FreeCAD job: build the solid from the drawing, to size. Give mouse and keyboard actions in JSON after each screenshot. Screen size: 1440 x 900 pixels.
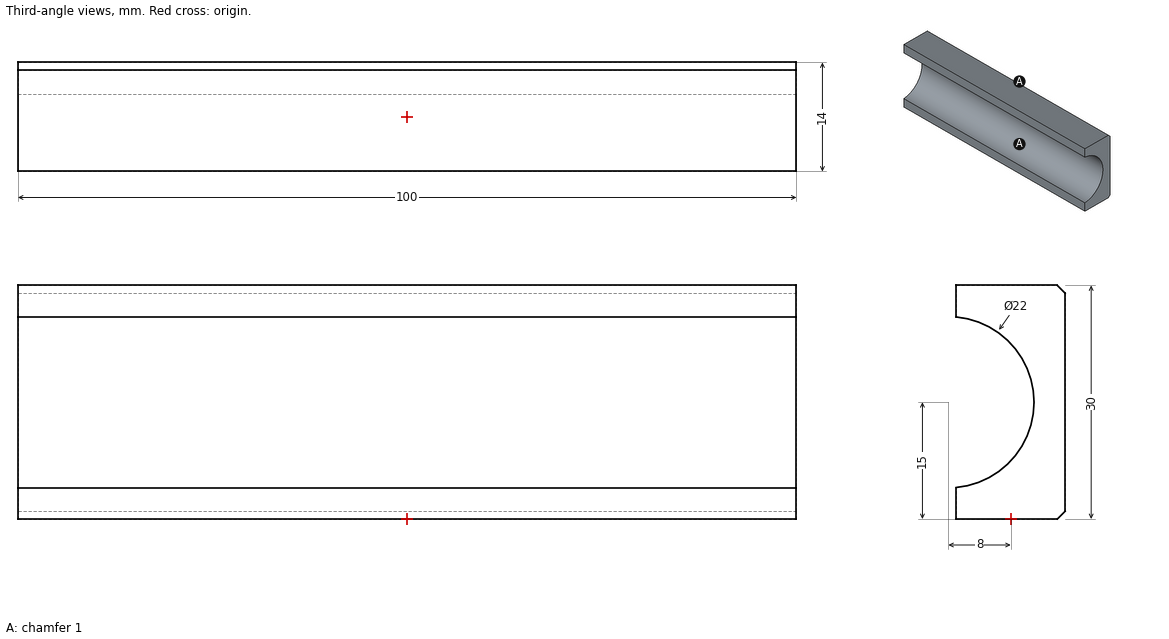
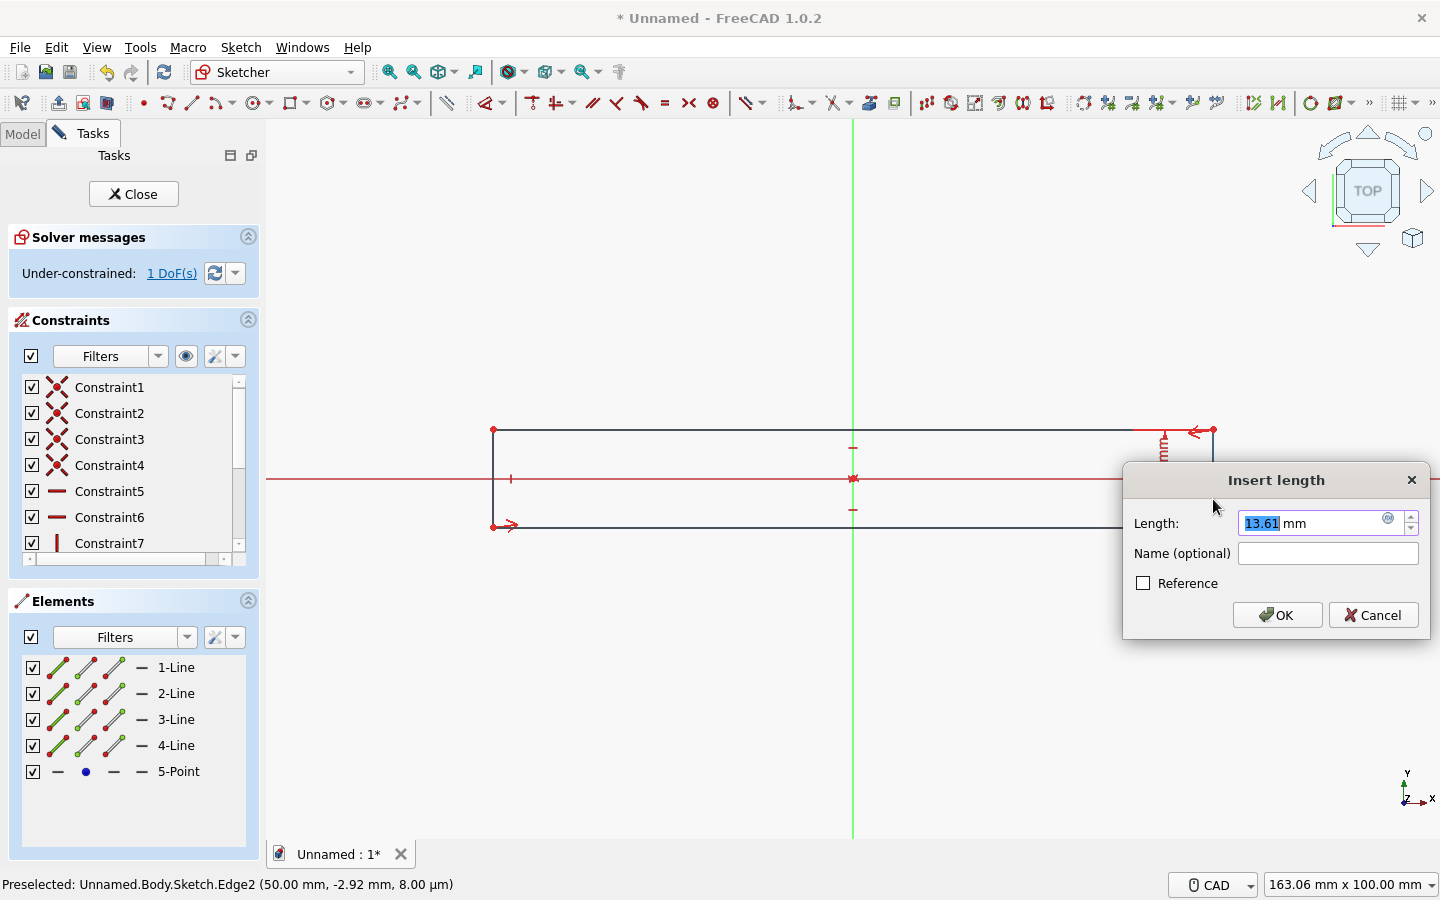
{"action": "type", "text": "14"}
{"action": "key", "text": "Return"}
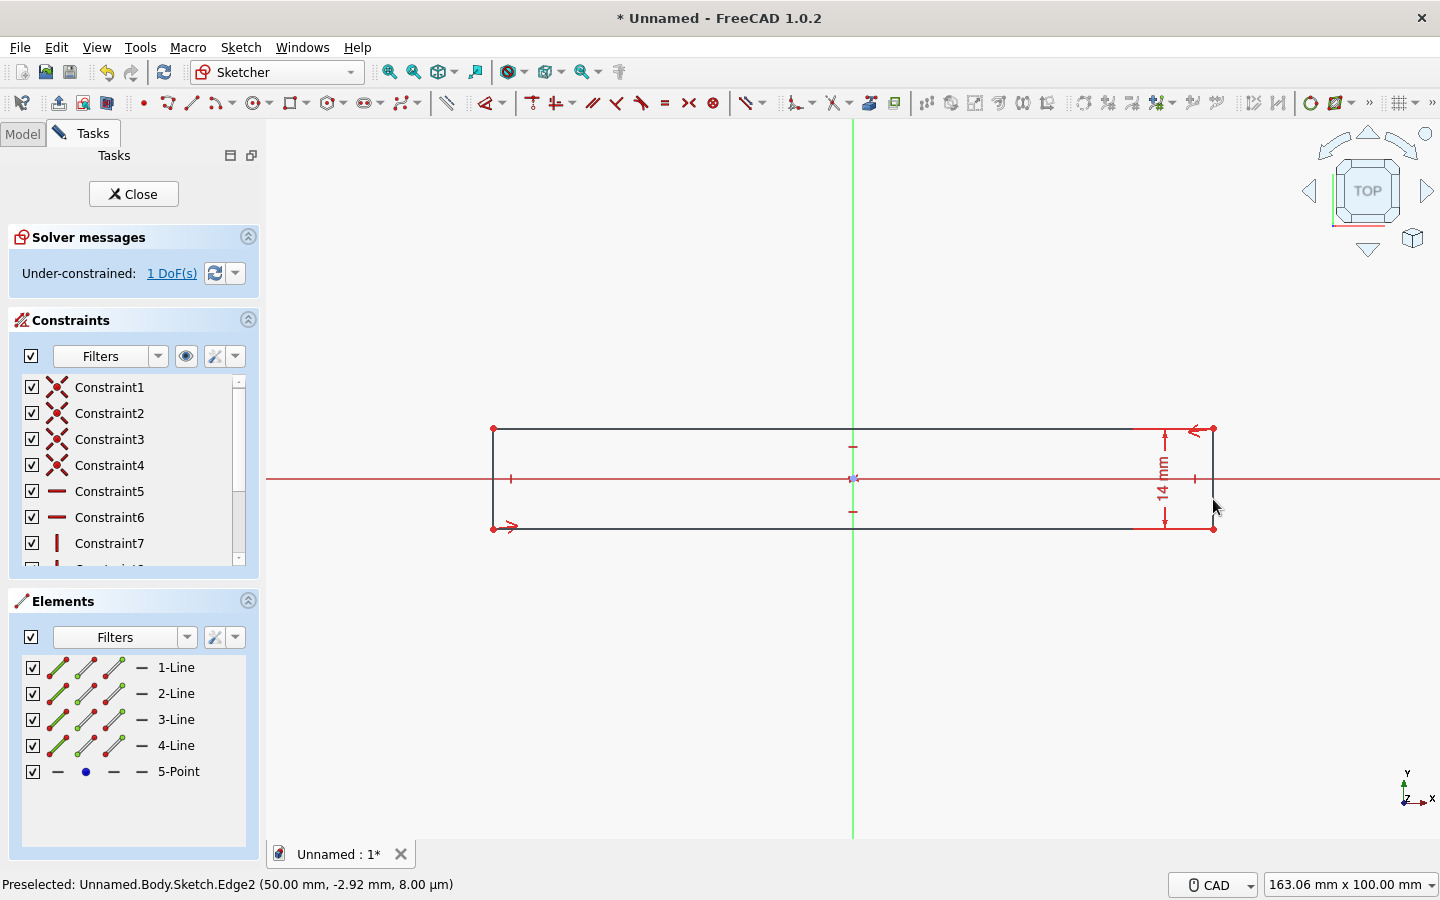
{"action": "left_click", "coordinate": [709, 529]}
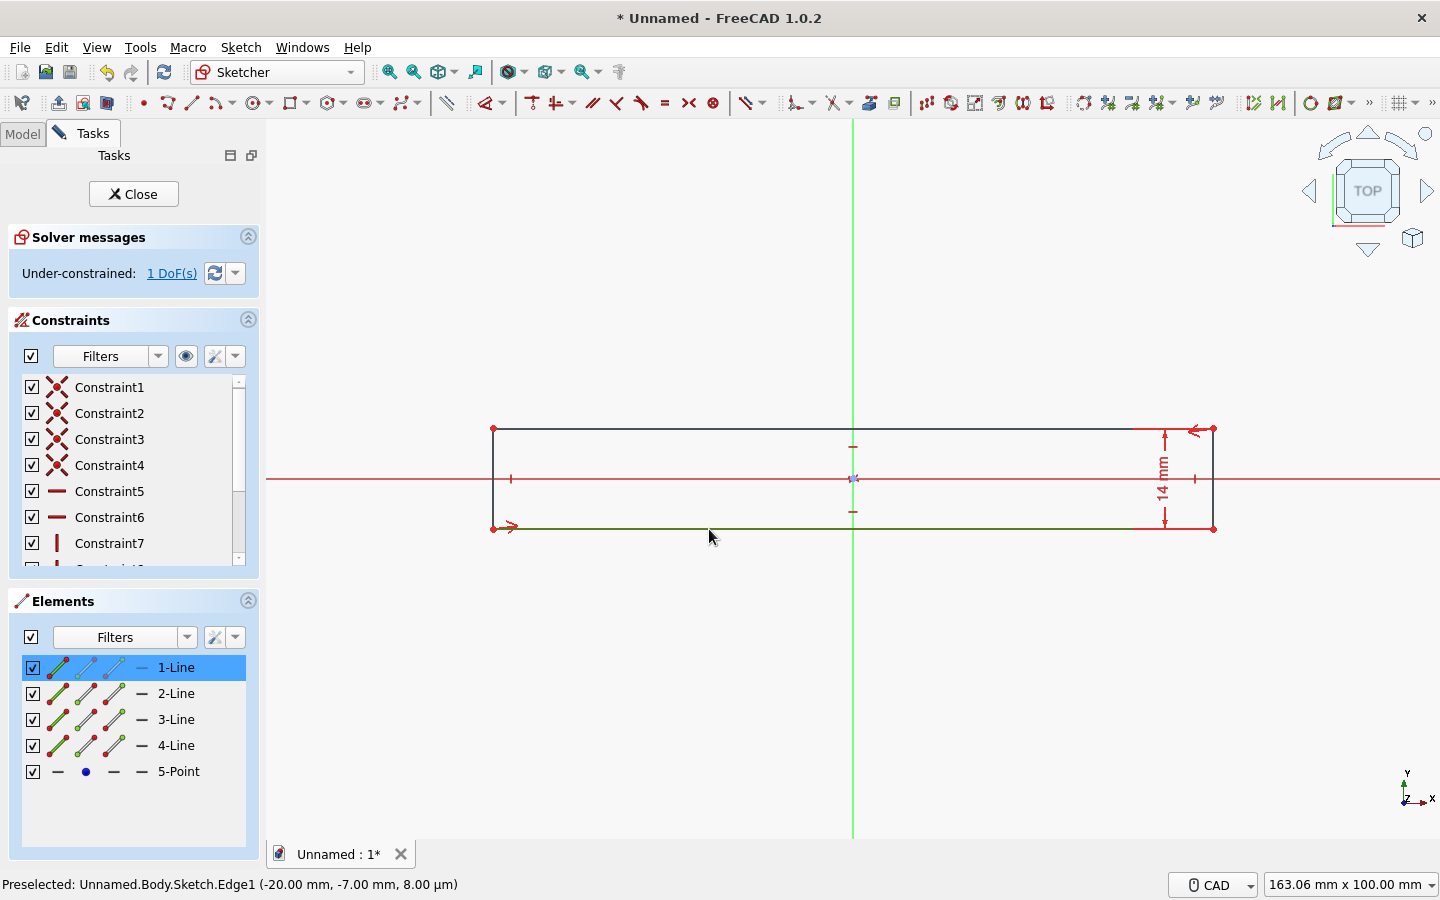
{"action": "left_click", "coordinate": [504, 104]}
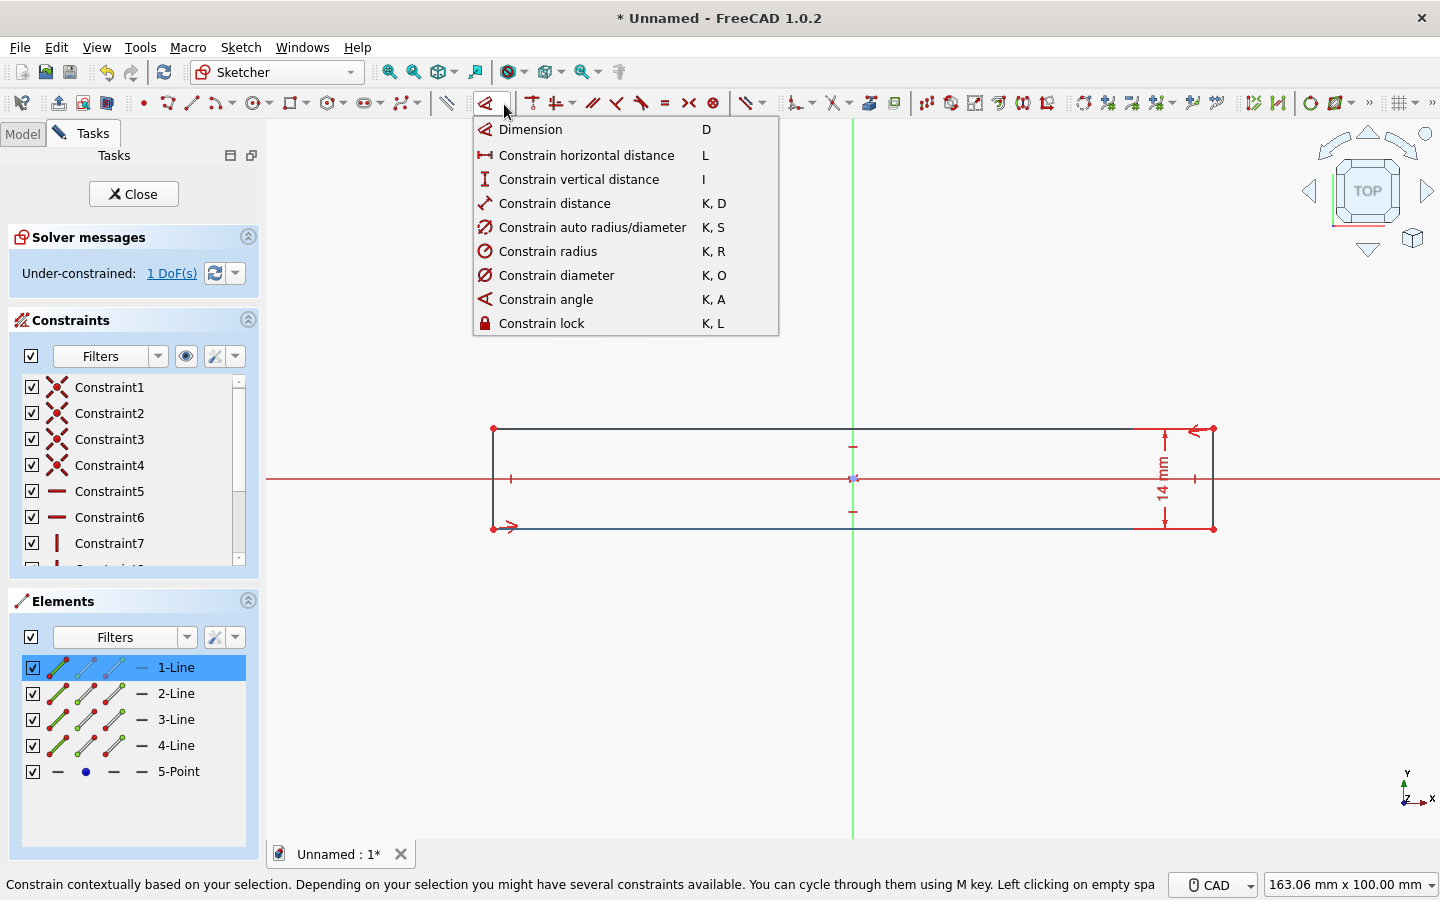
{"action": "left_click", "coordinate": [626, 155]}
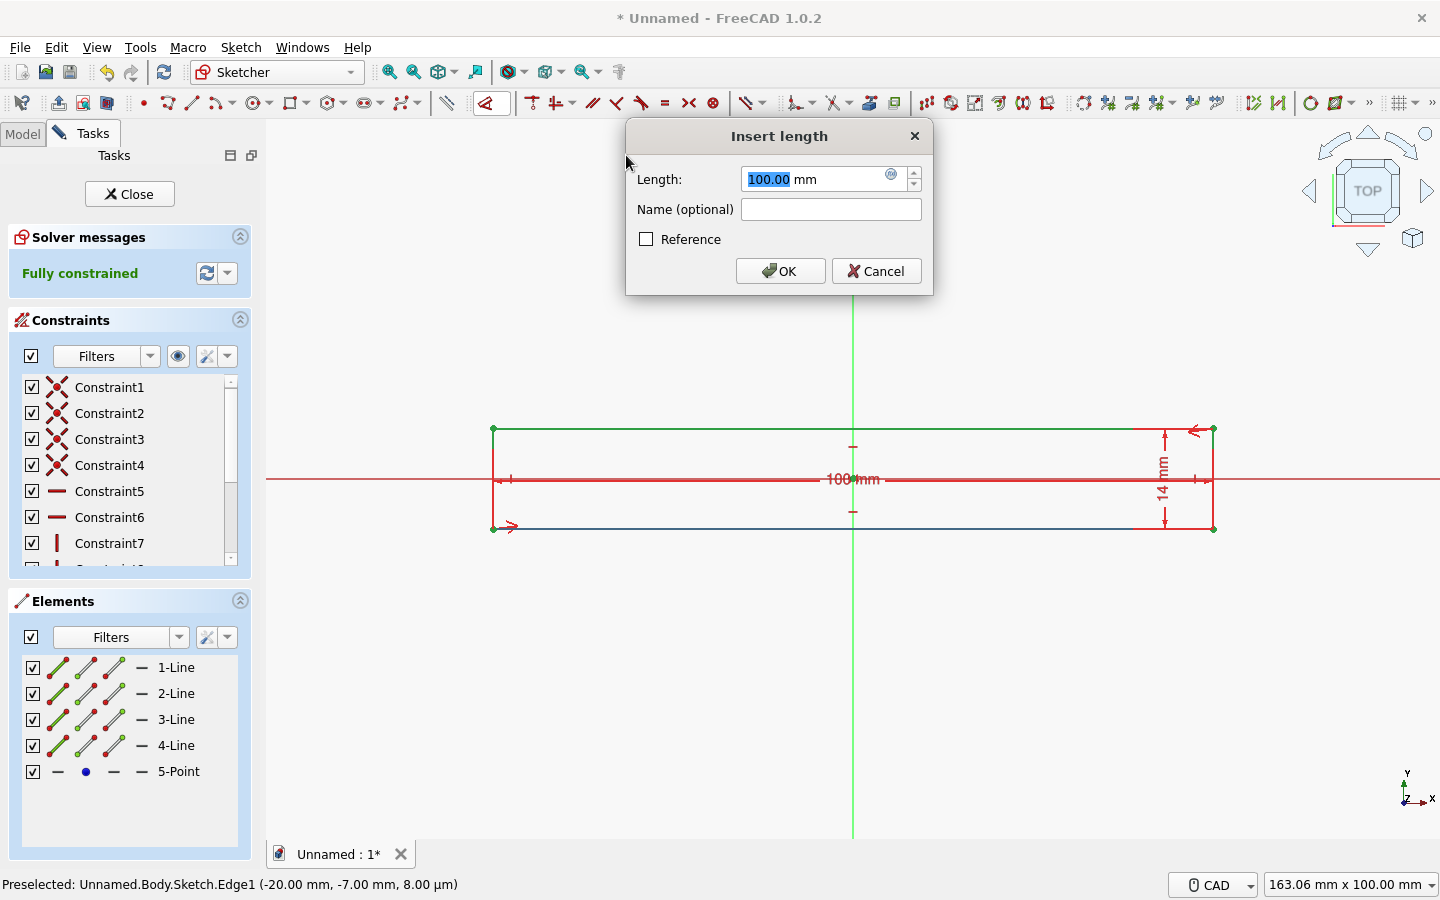
{"action": "type", "text": "100"}
{"action": "key", "text": "Return"}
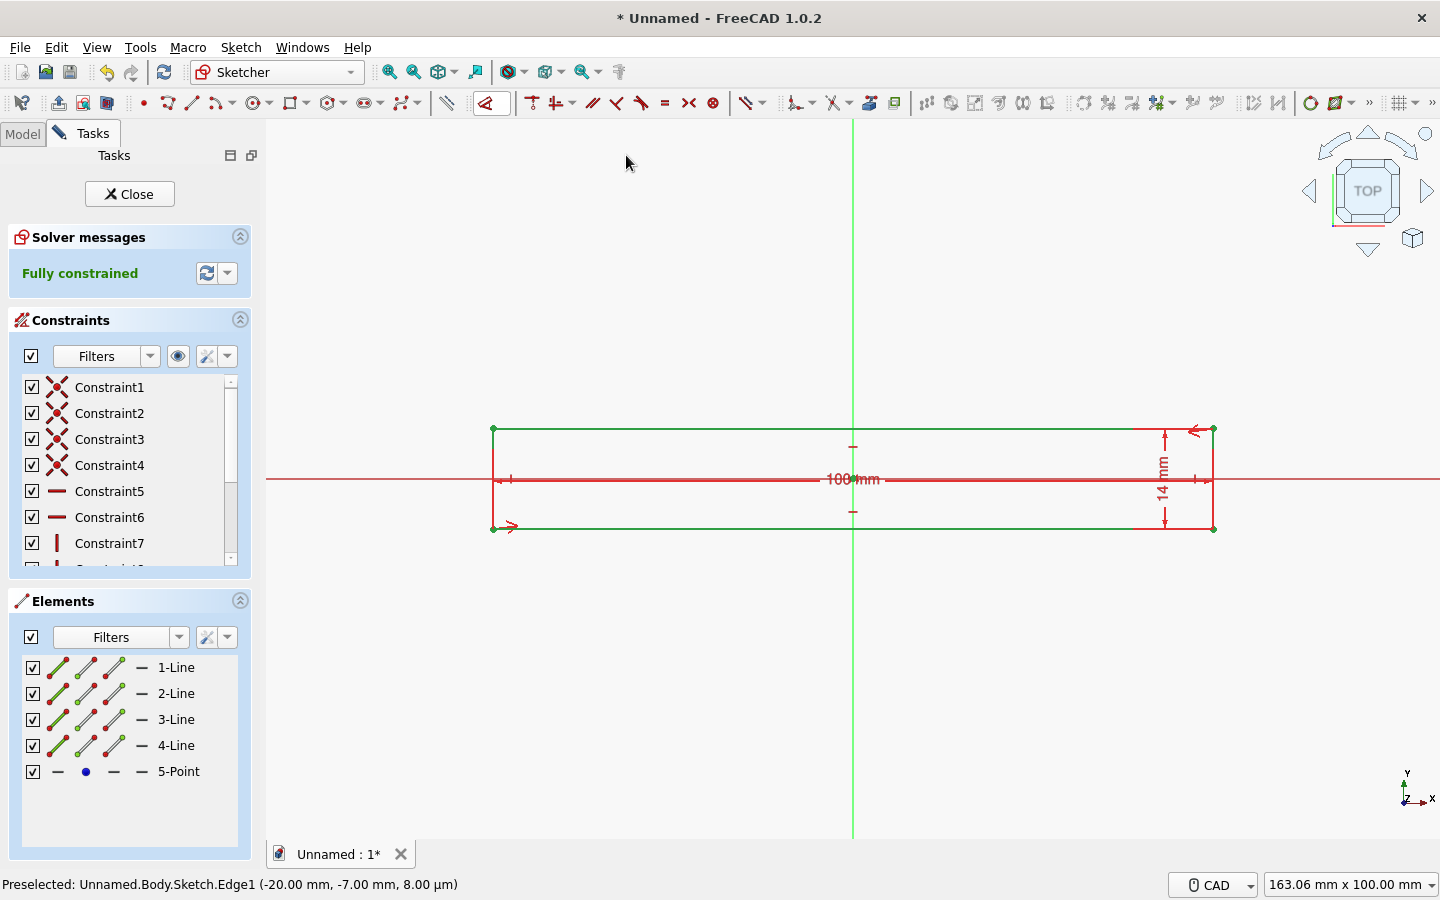
{"action": "left_click", "coordinate": [130, 194]}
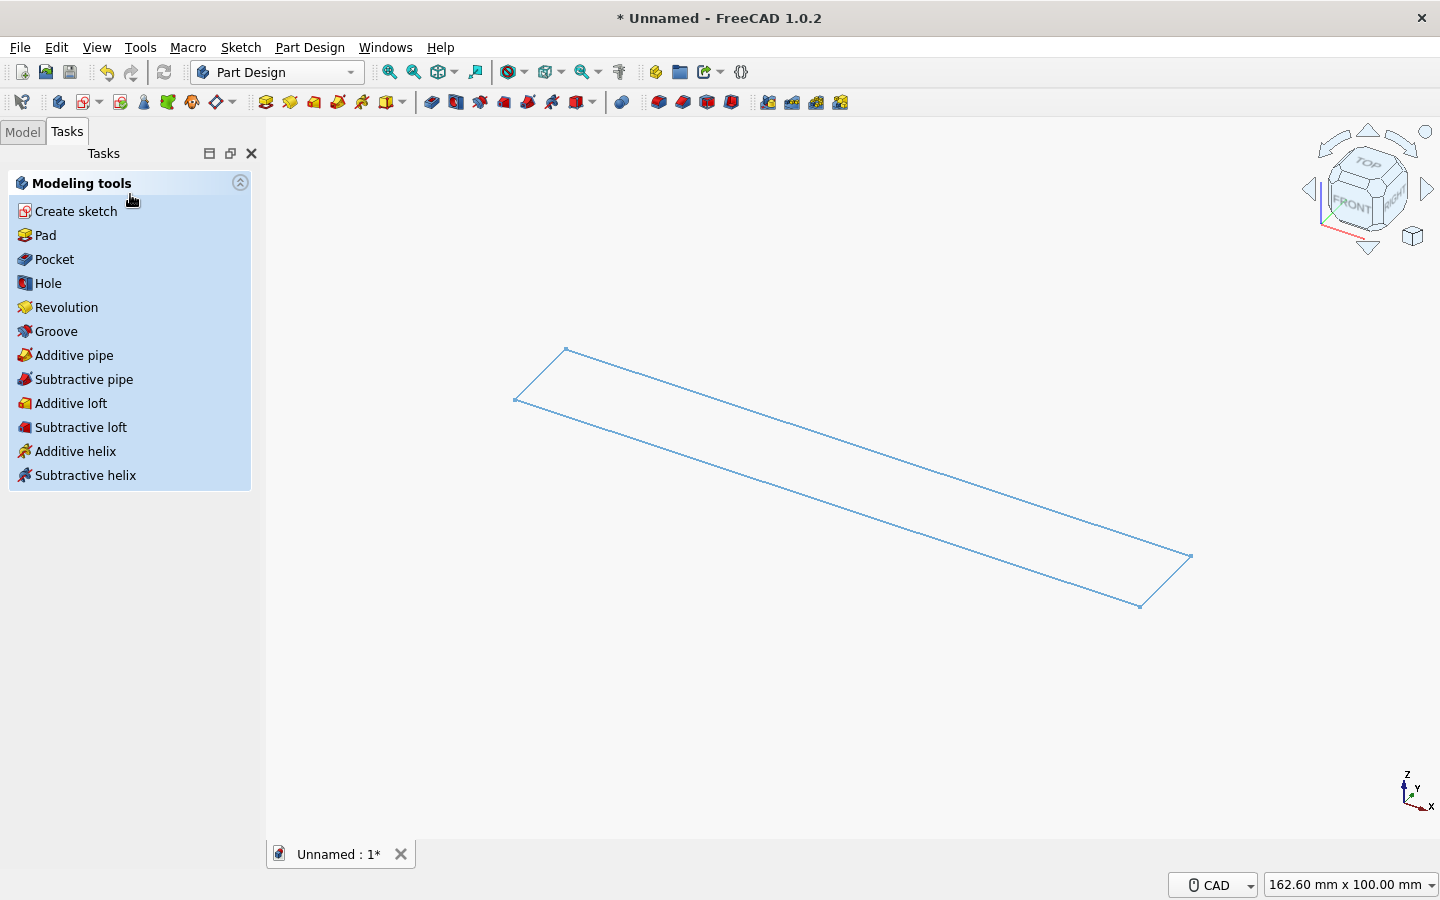
{"action": "left_click", "coordinate": [266, 102]}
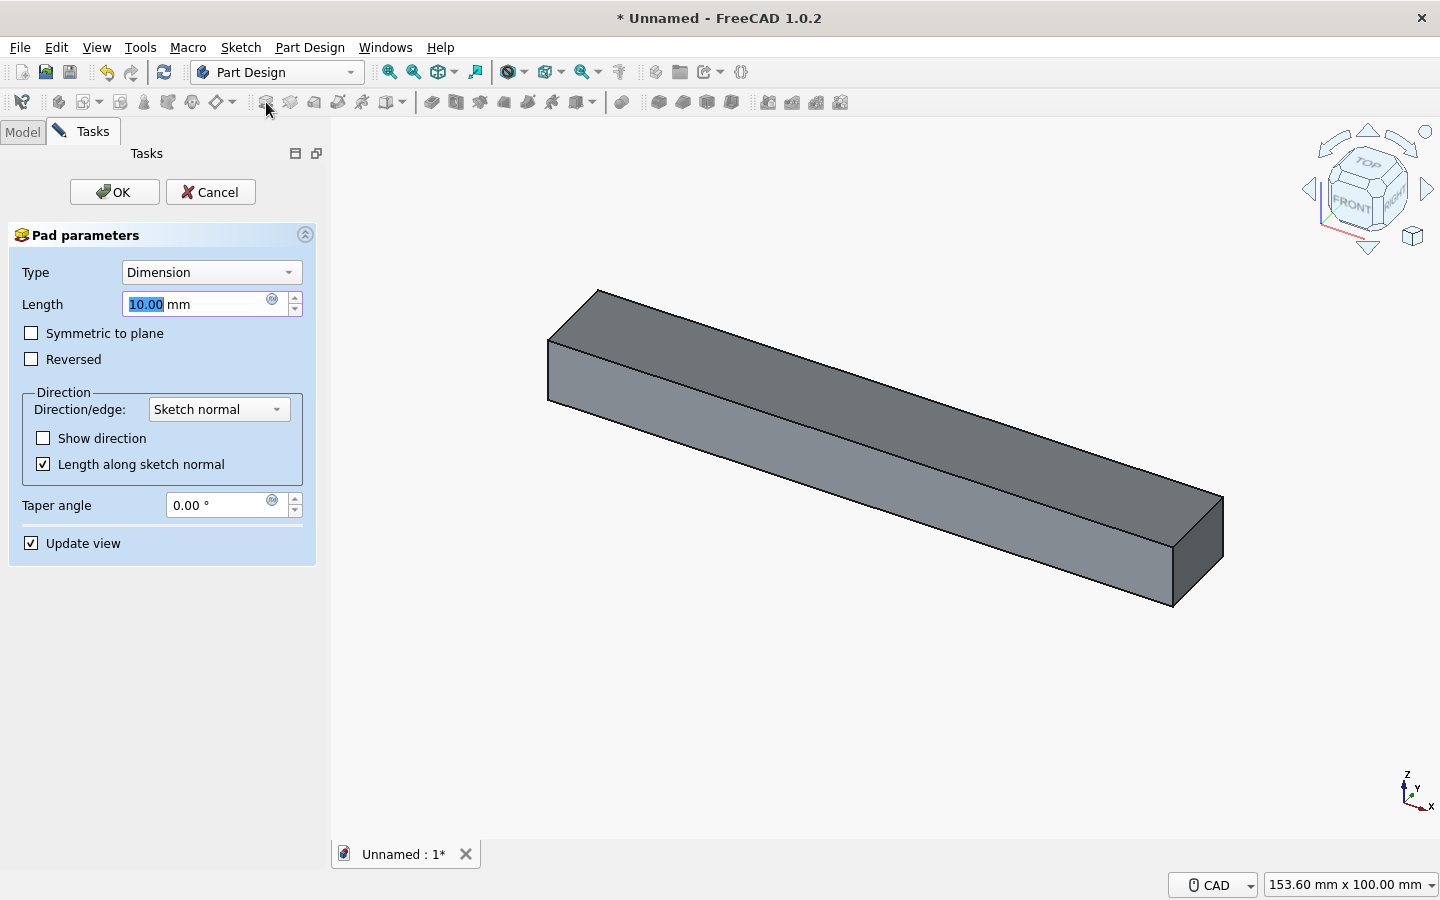
{"action": "type", "text": "30"}
{"action": "key", "text": "Tab"}